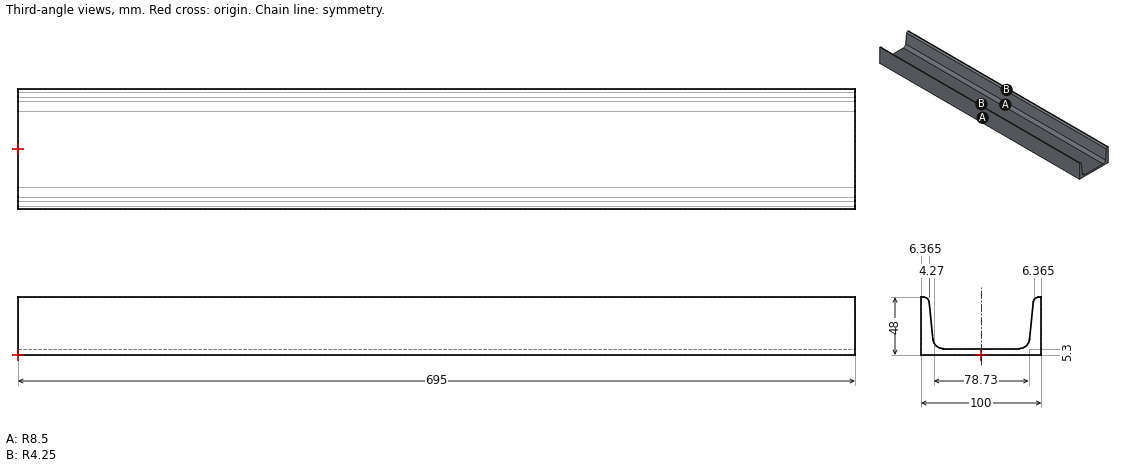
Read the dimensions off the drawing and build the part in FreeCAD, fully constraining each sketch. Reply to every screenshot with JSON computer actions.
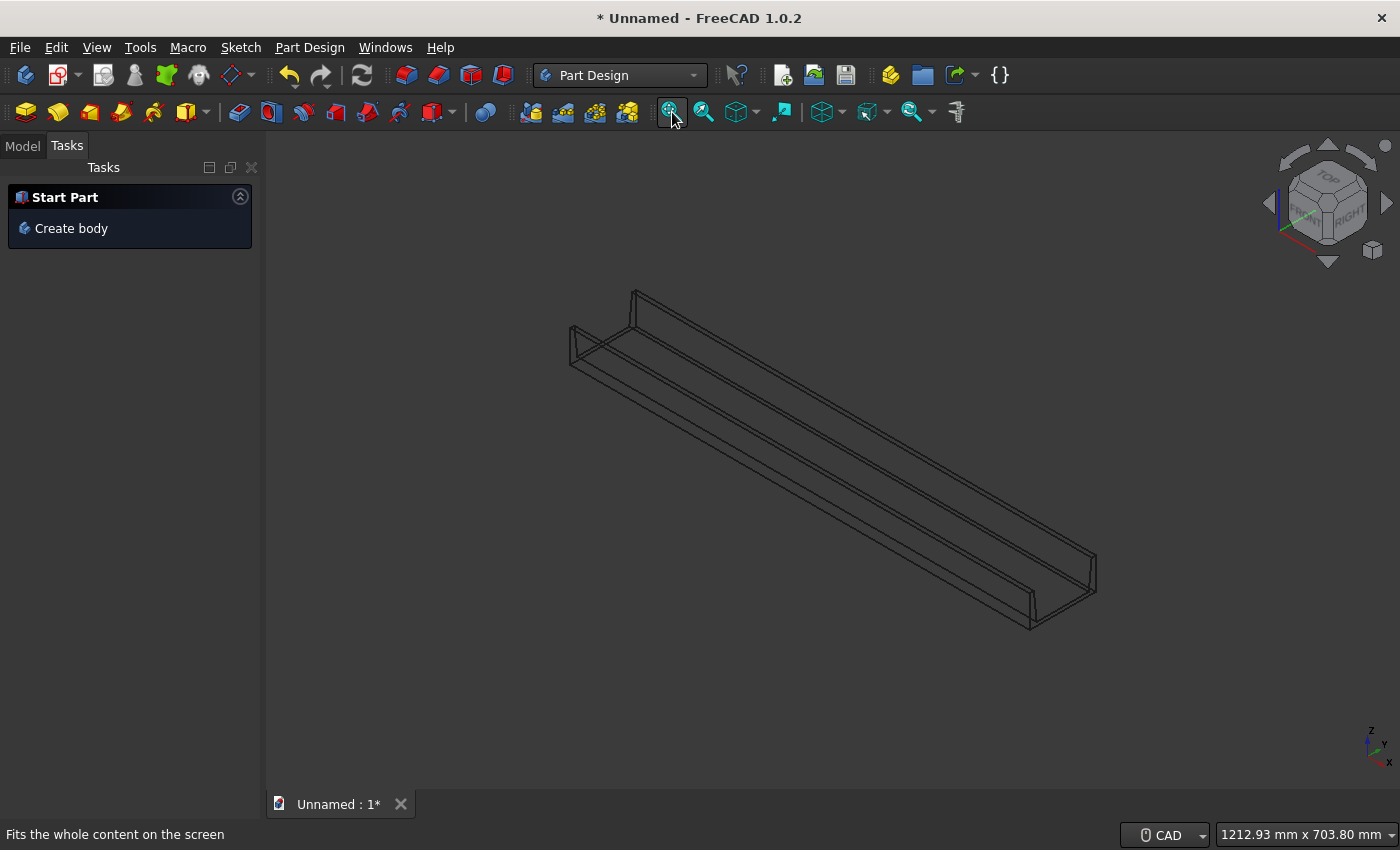
{"action": "left_click", "coordinate": [807, 488]}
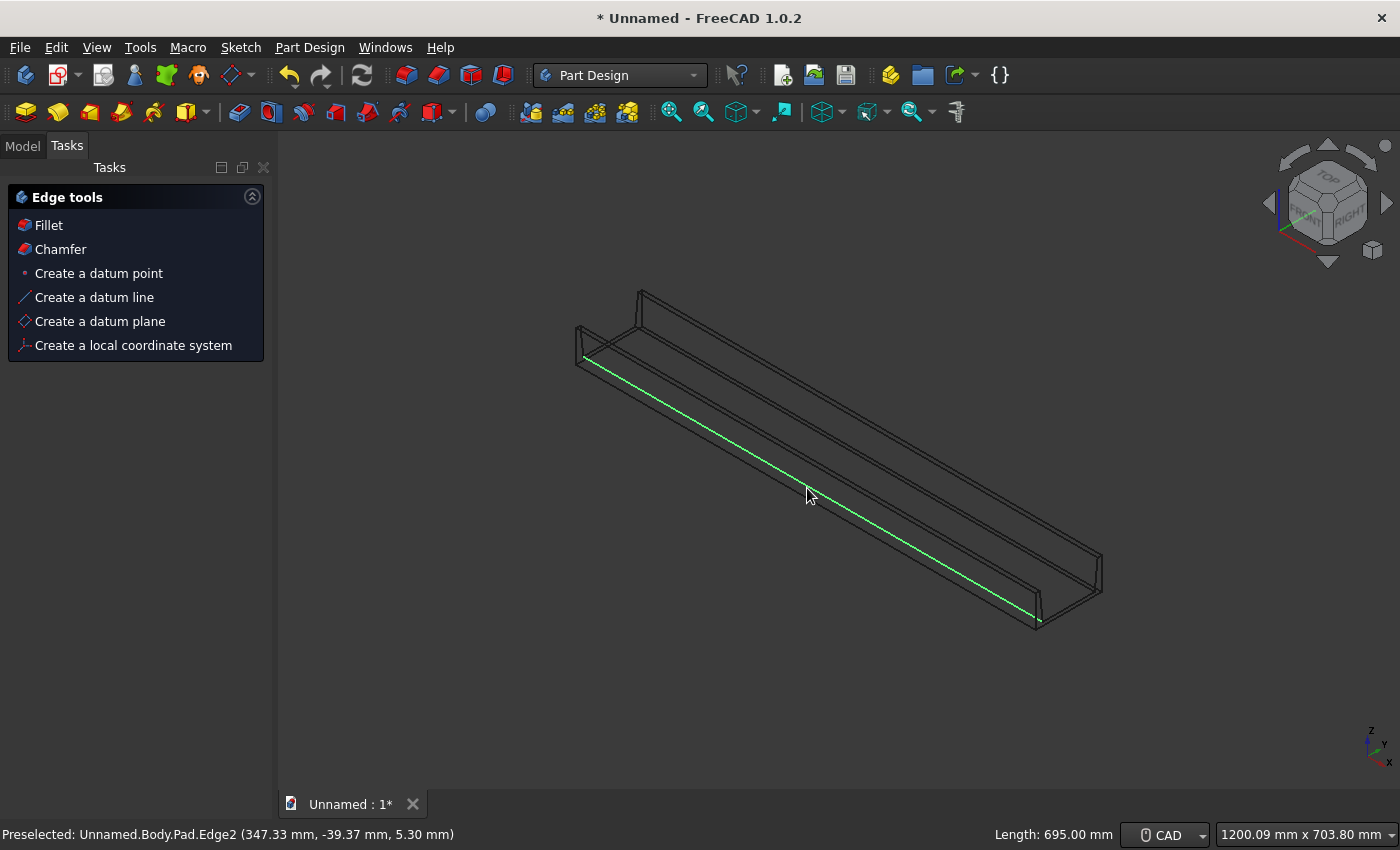
{"action": "left_click", "coordinate": [865, 458], "text": "ctrl"}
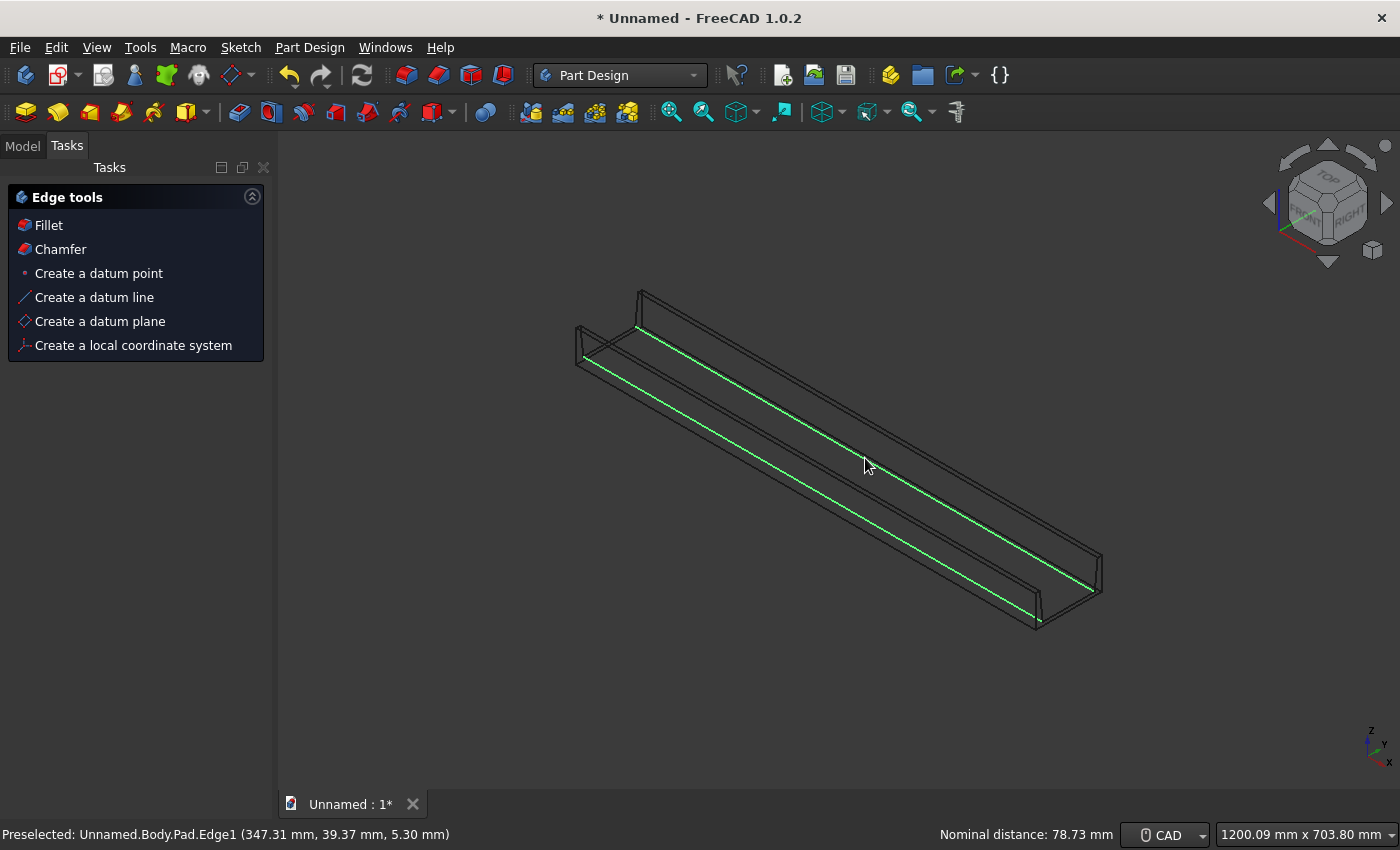
{"action": "key", "text": "v 1"}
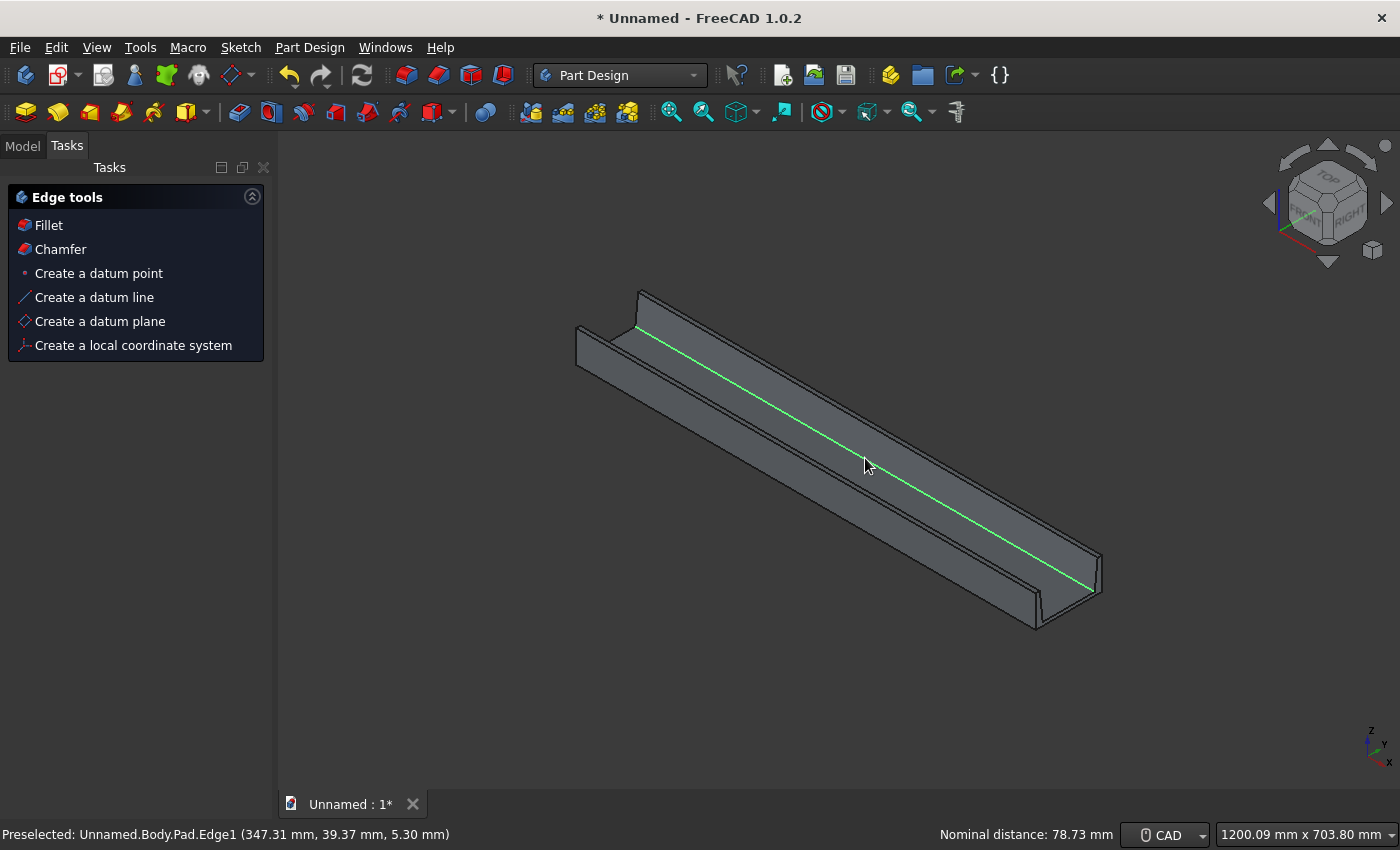
{"action": "left_click", "coordinate": [408, 76]}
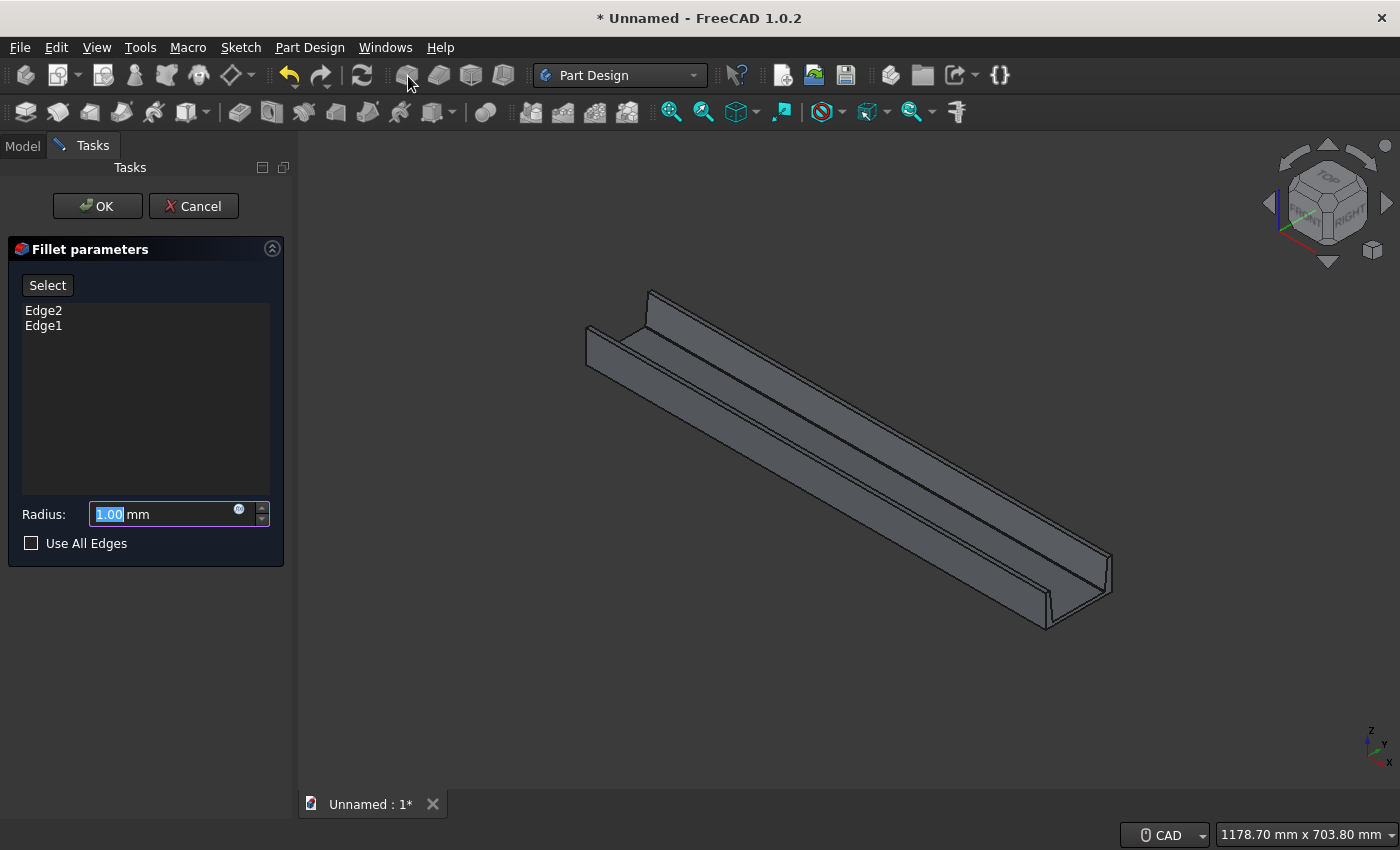
{"action": "type", "text": "8.5"}
{"action": "key", "text": "Tab"}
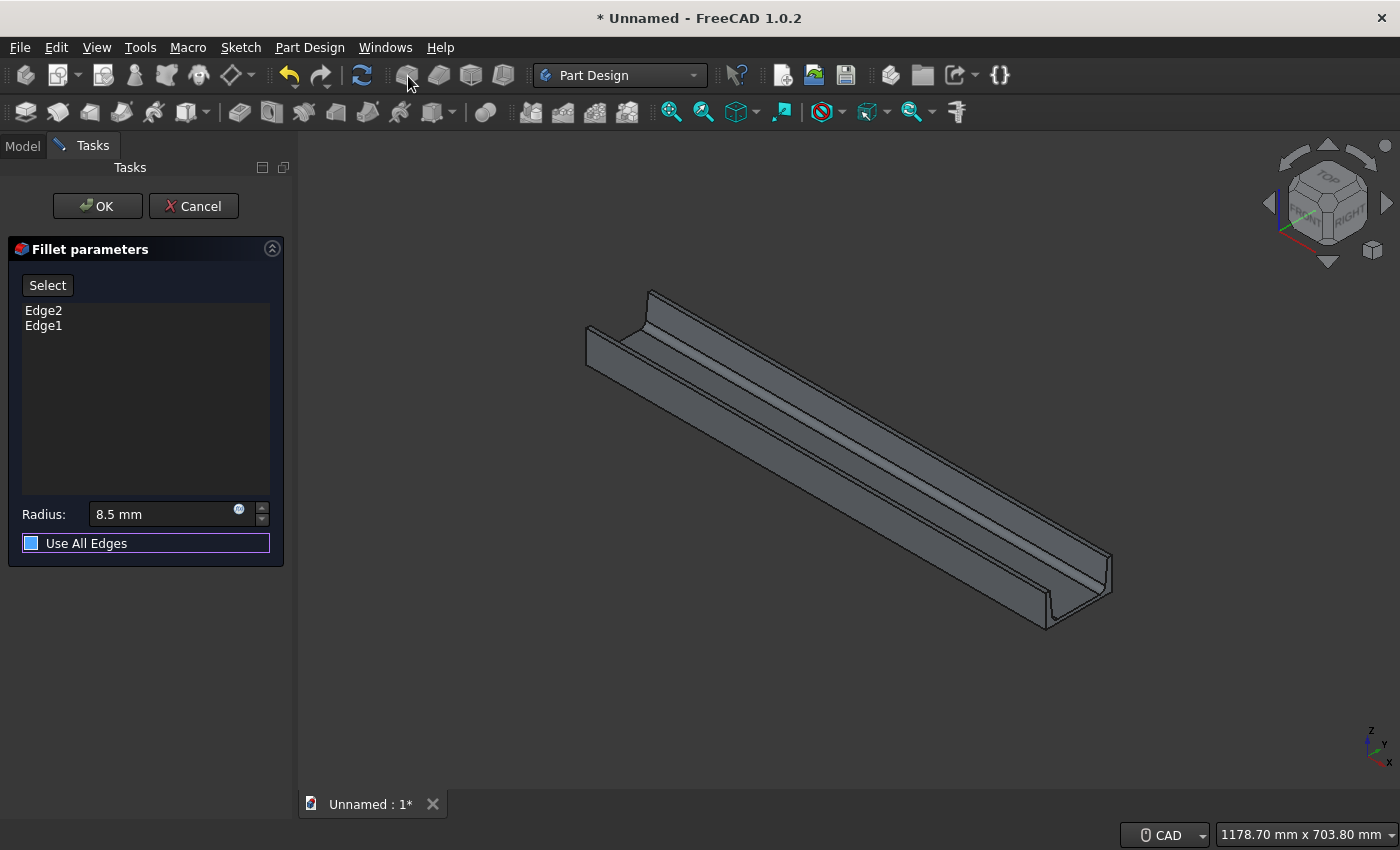
{"action": "left_click", "coordinate": [98, 206]}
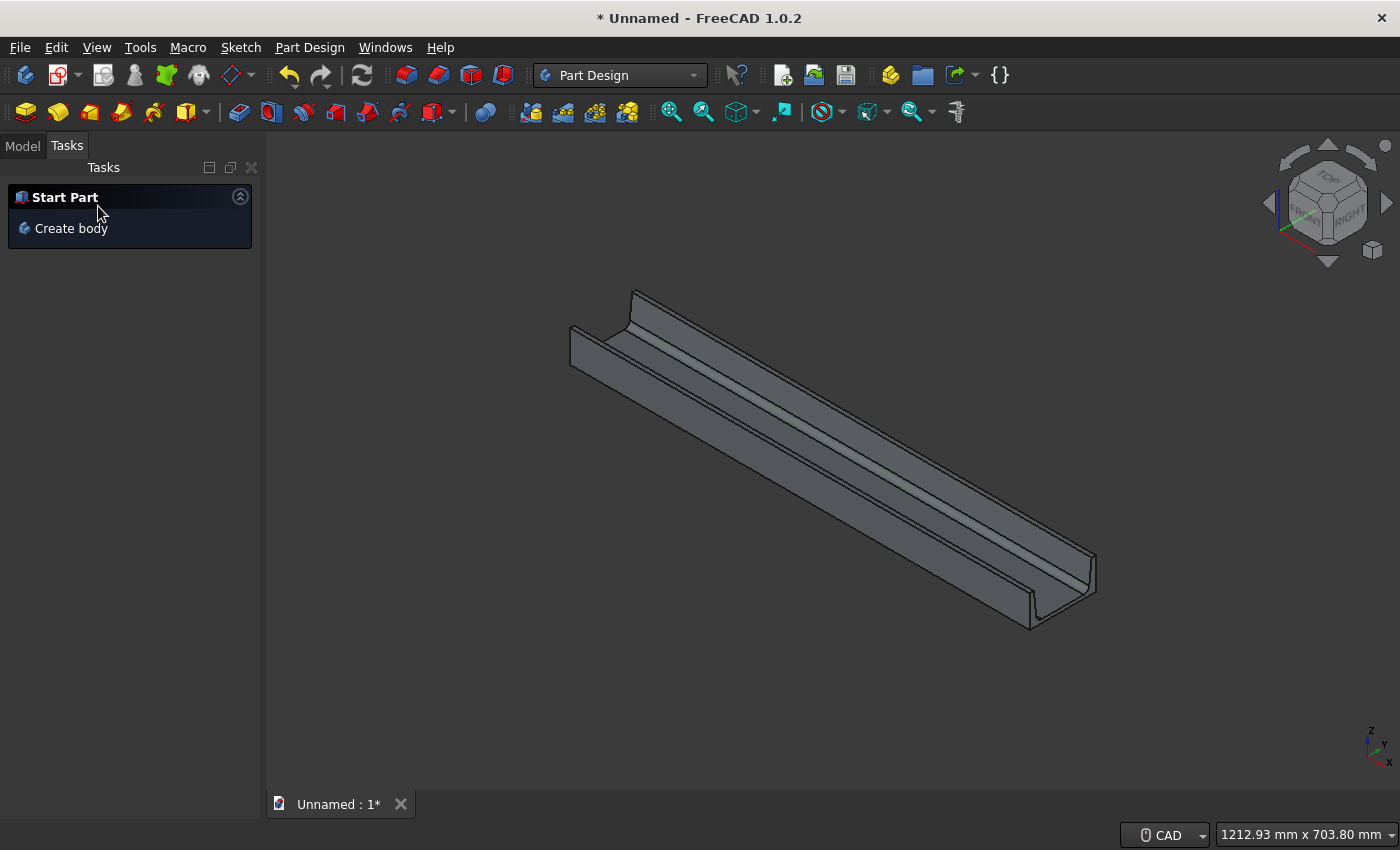
{"action": "left_click", "coordinate": [862, 424]}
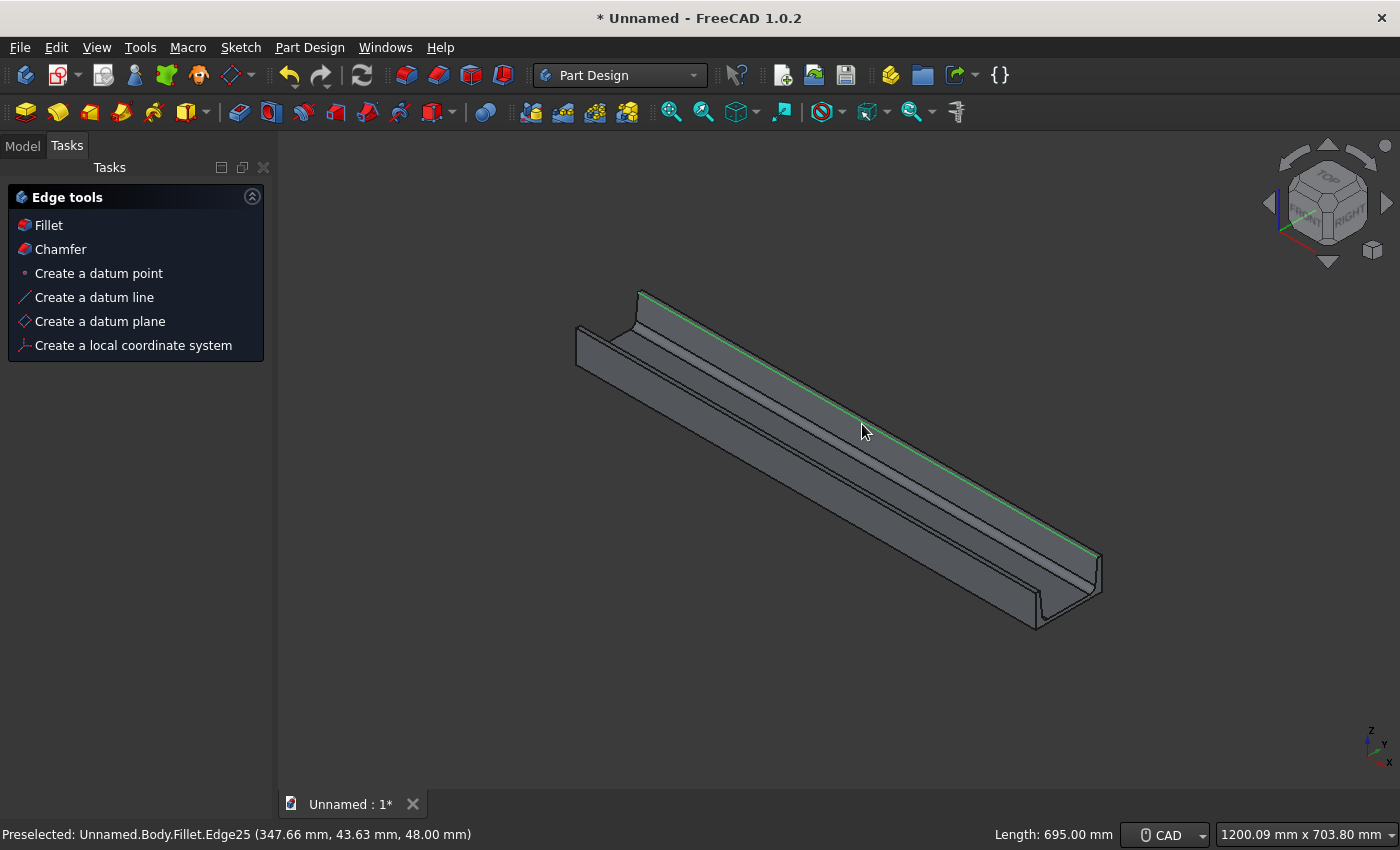
{"action": "key", "text": "2"}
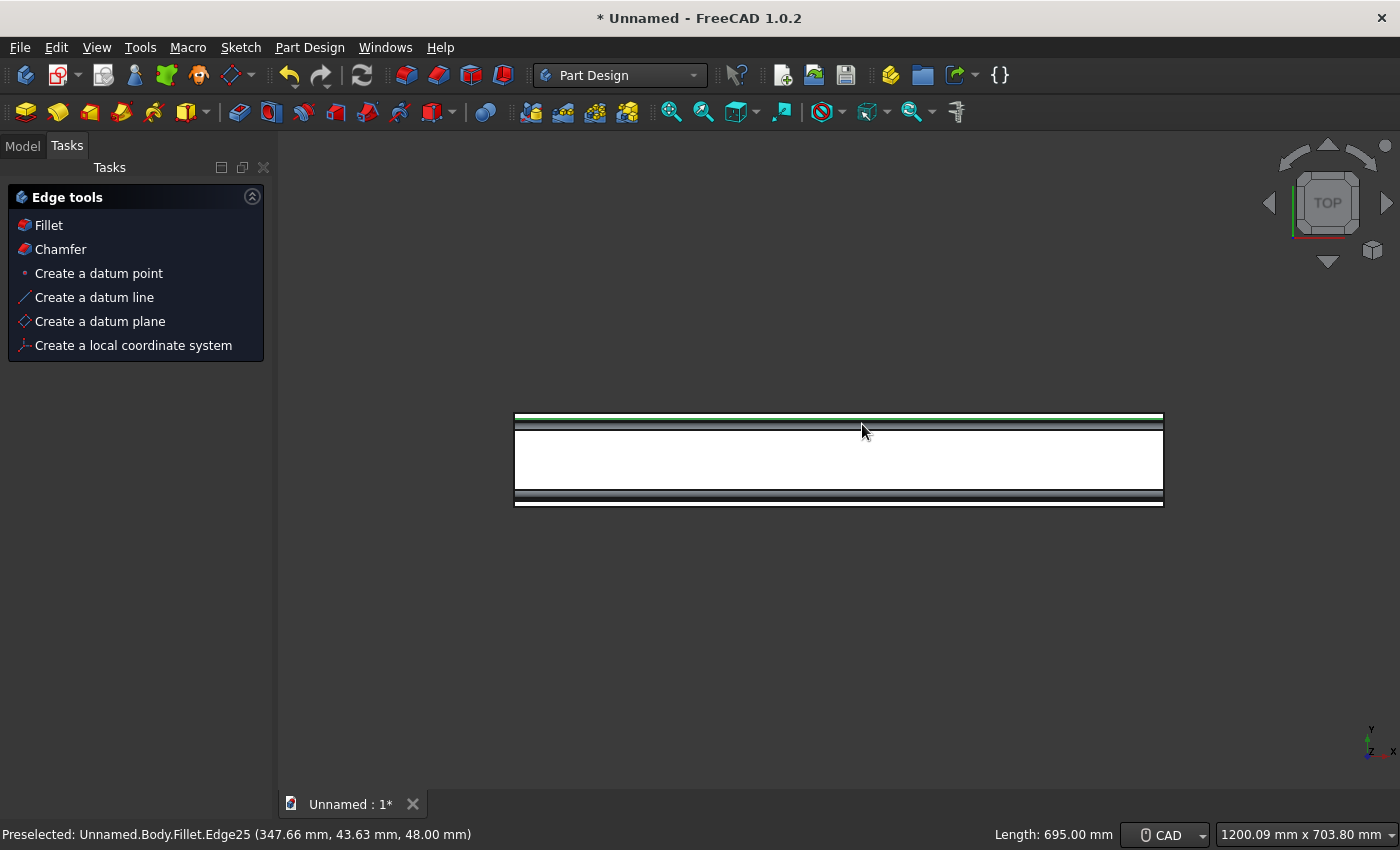
{"action": "left_click", "coordinate": [839, 500], "text": "ctrl"}